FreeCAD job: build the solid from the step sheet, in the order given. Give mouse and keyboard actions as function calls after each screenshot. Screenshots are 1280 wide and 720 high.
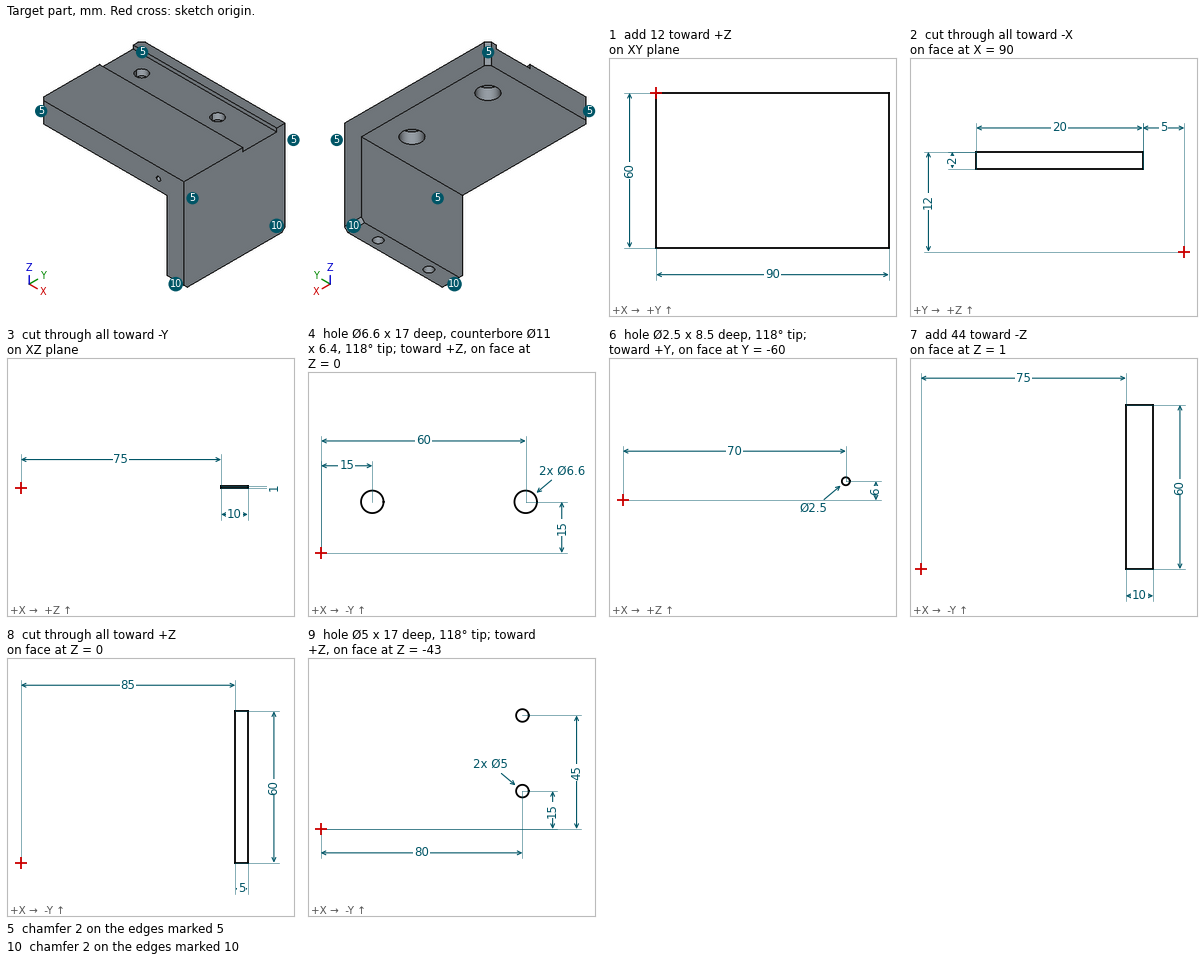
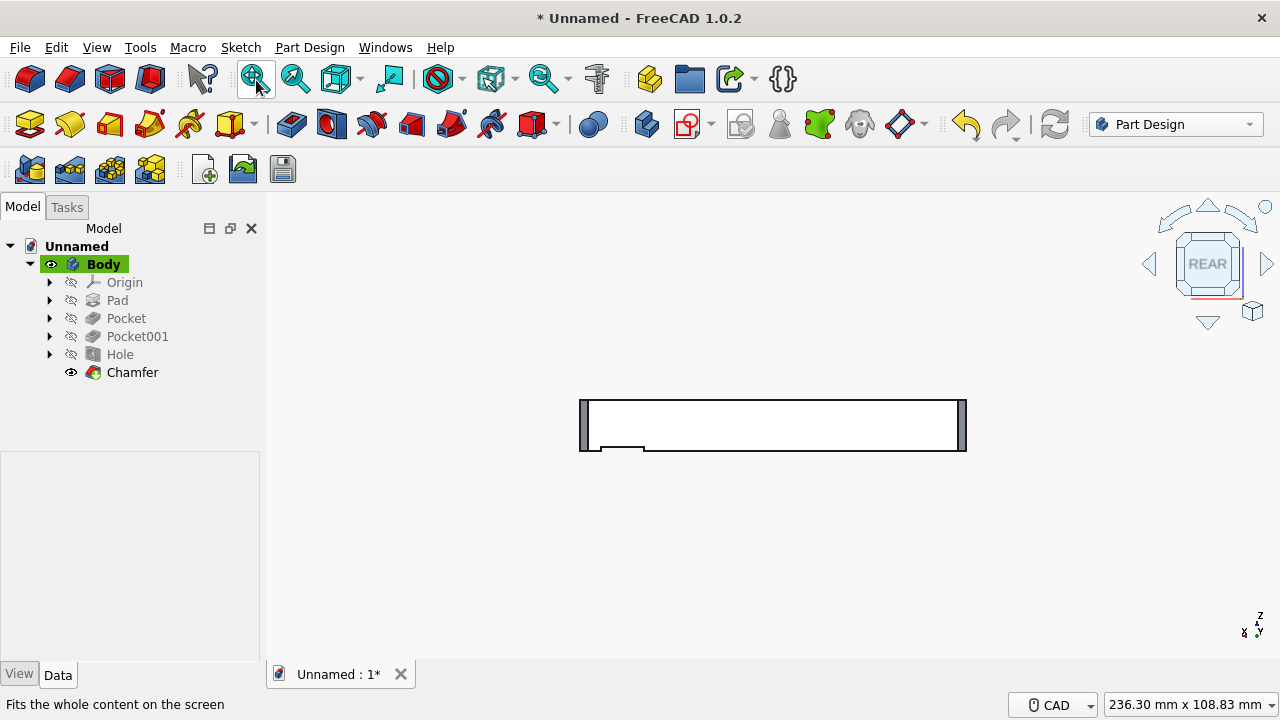
key(0)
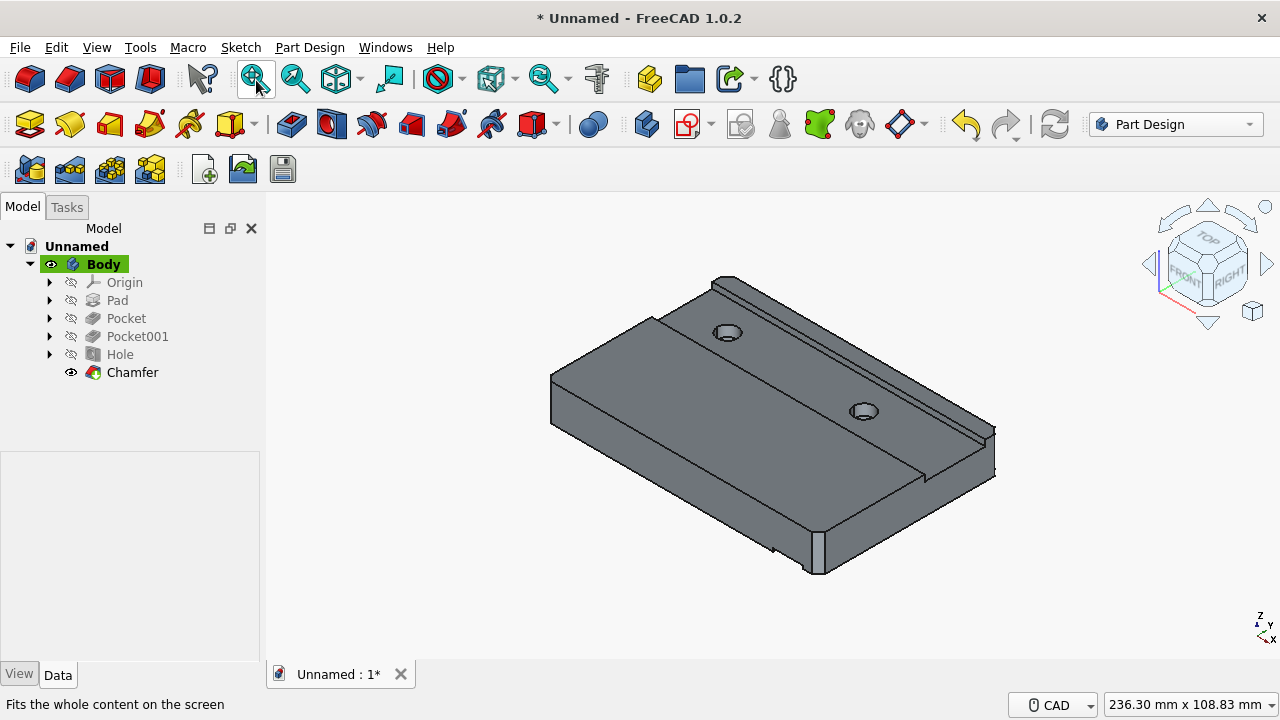
click(757, 520)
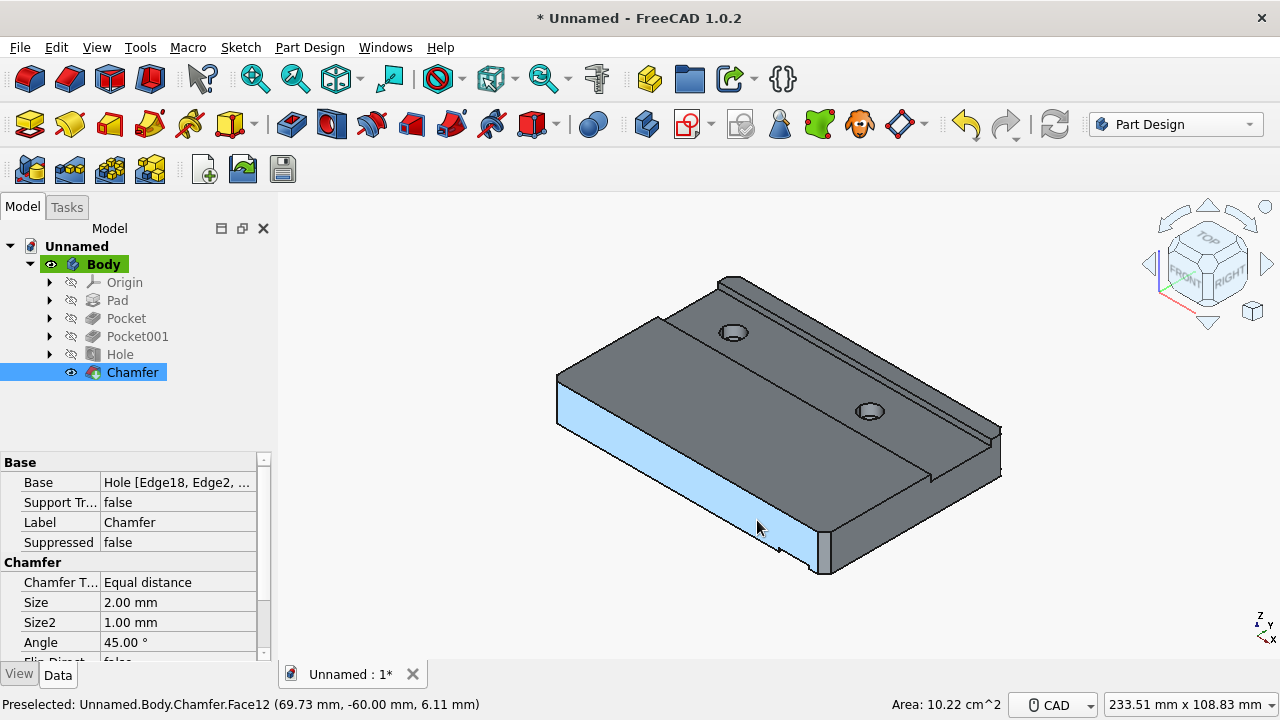
click(688, 124)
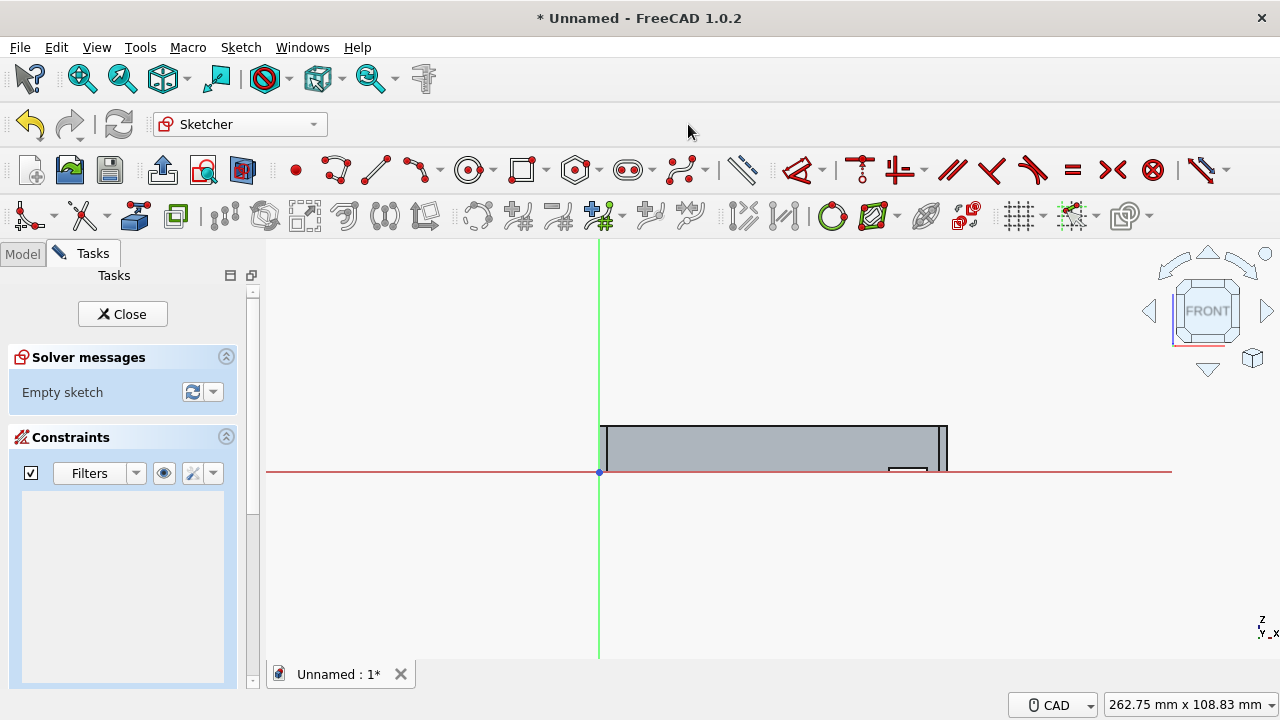
scroll(878, 449, up, 15)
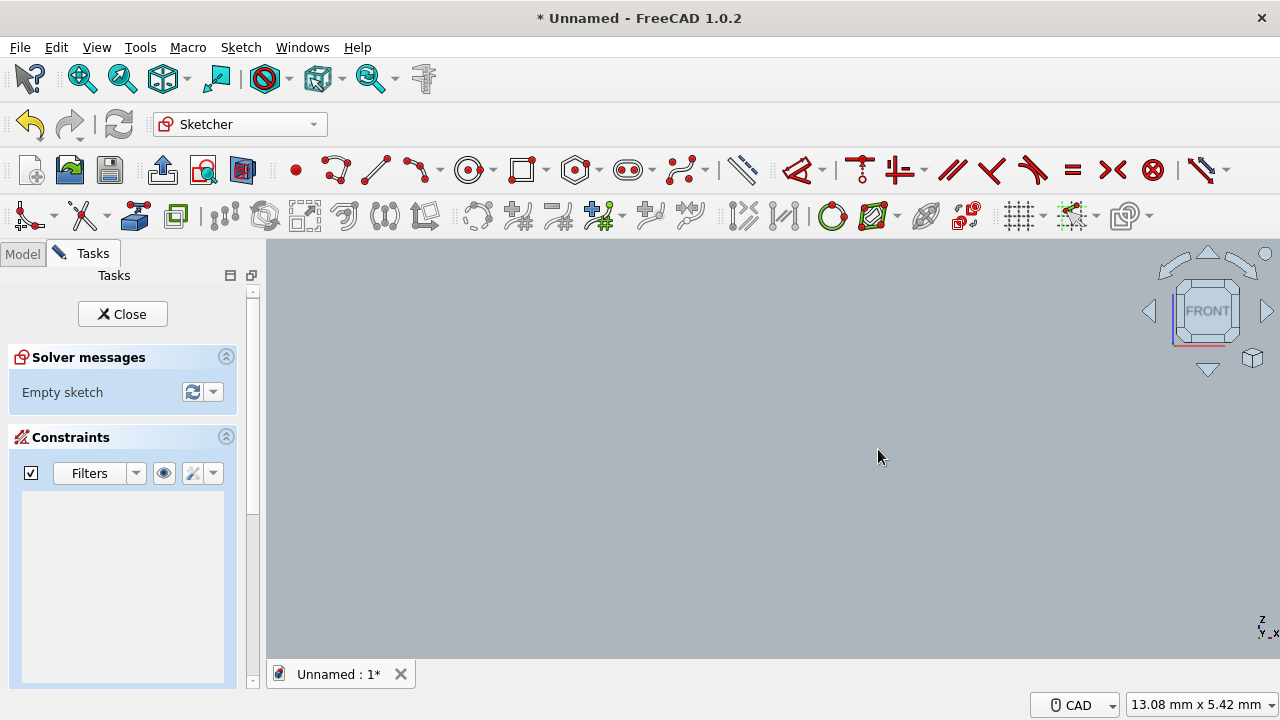
click(470, 170)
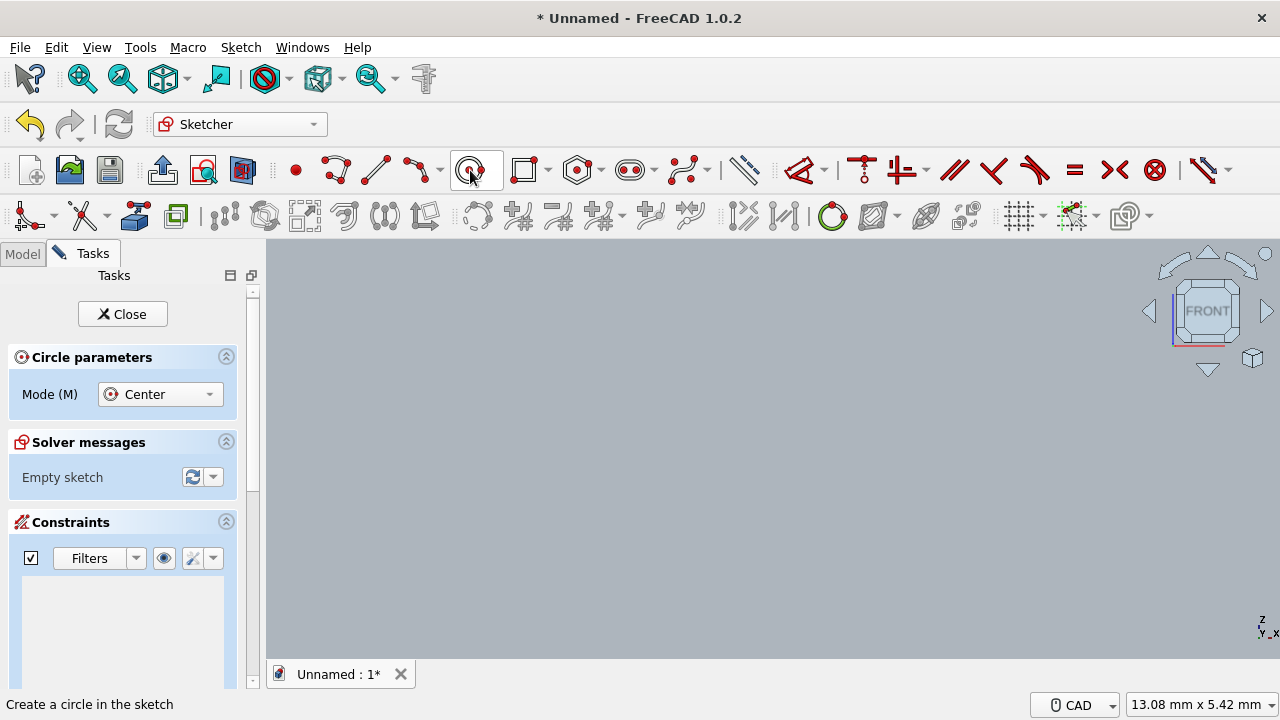
click(695, 439)
click(764, 371)
key(Escape)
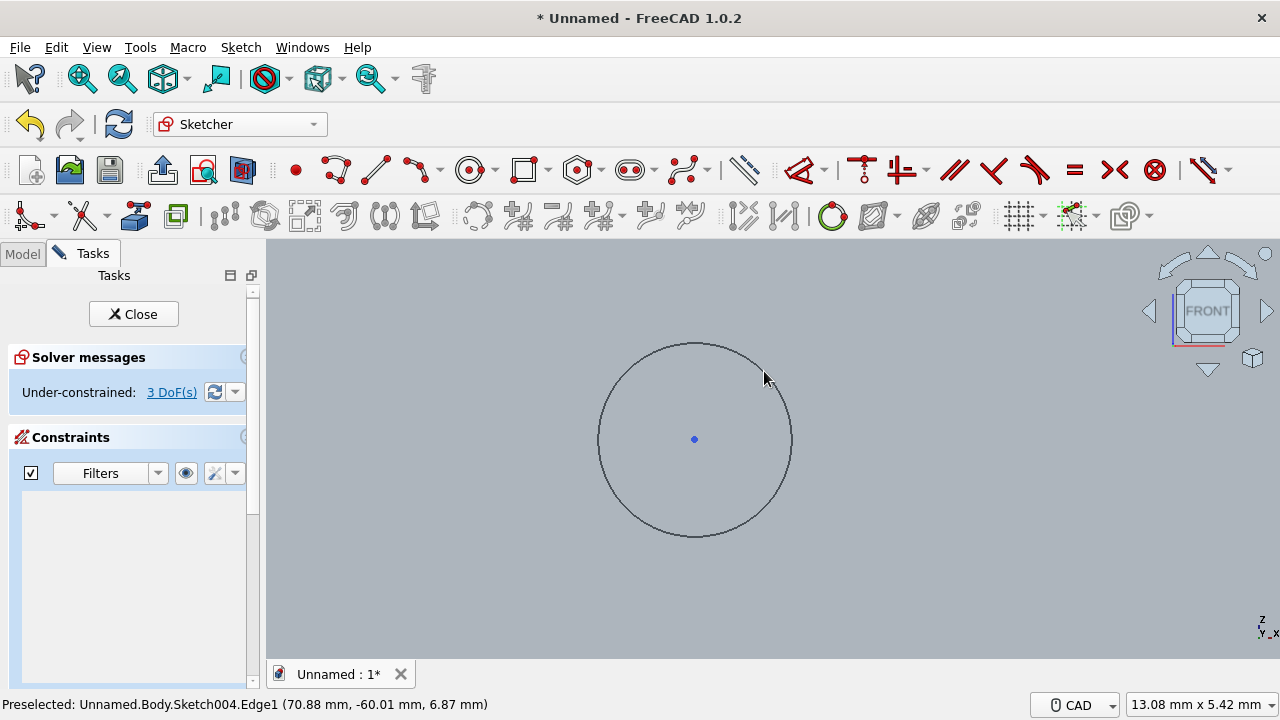
key(d)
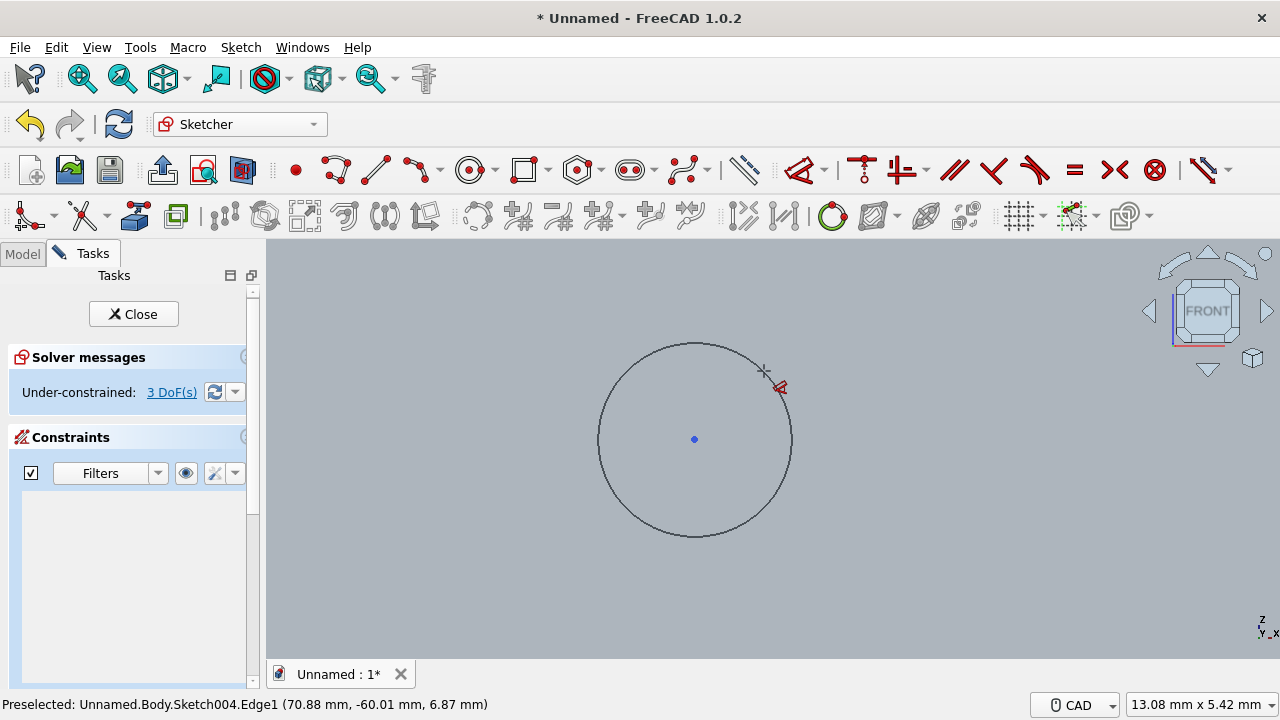
click(763, 371)
click(785, 348)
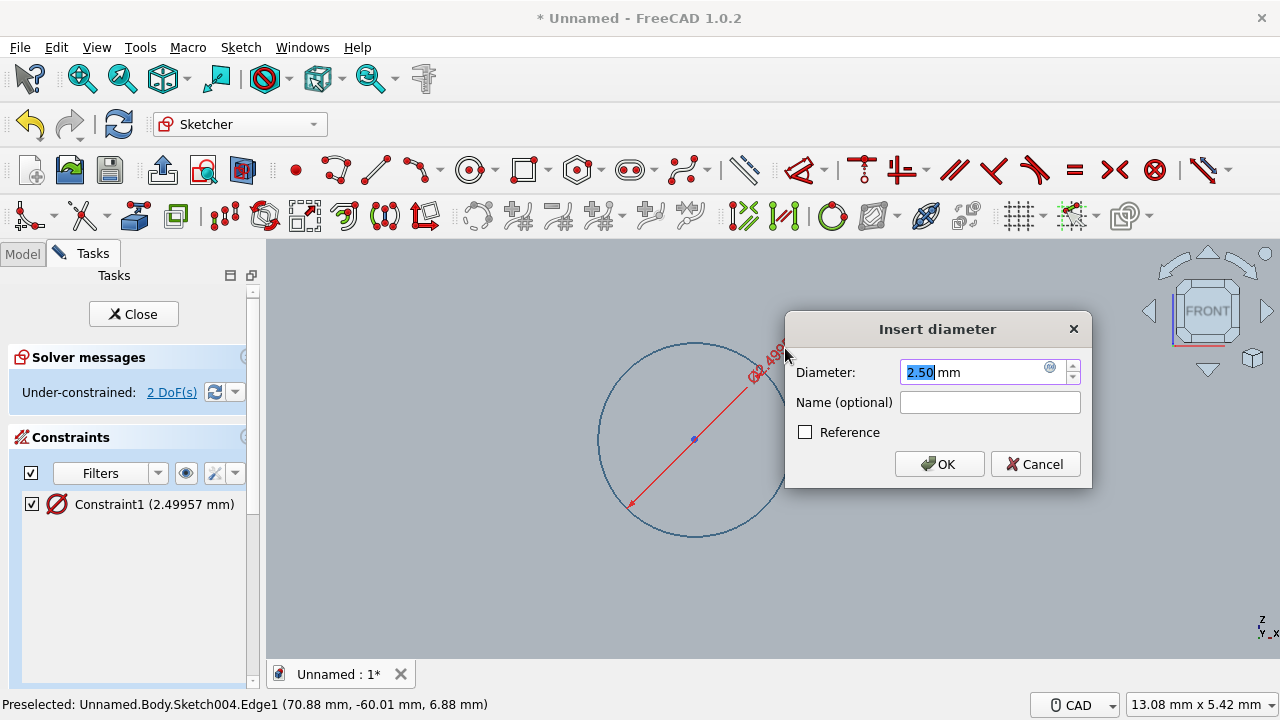
text(2.5)
key(Return)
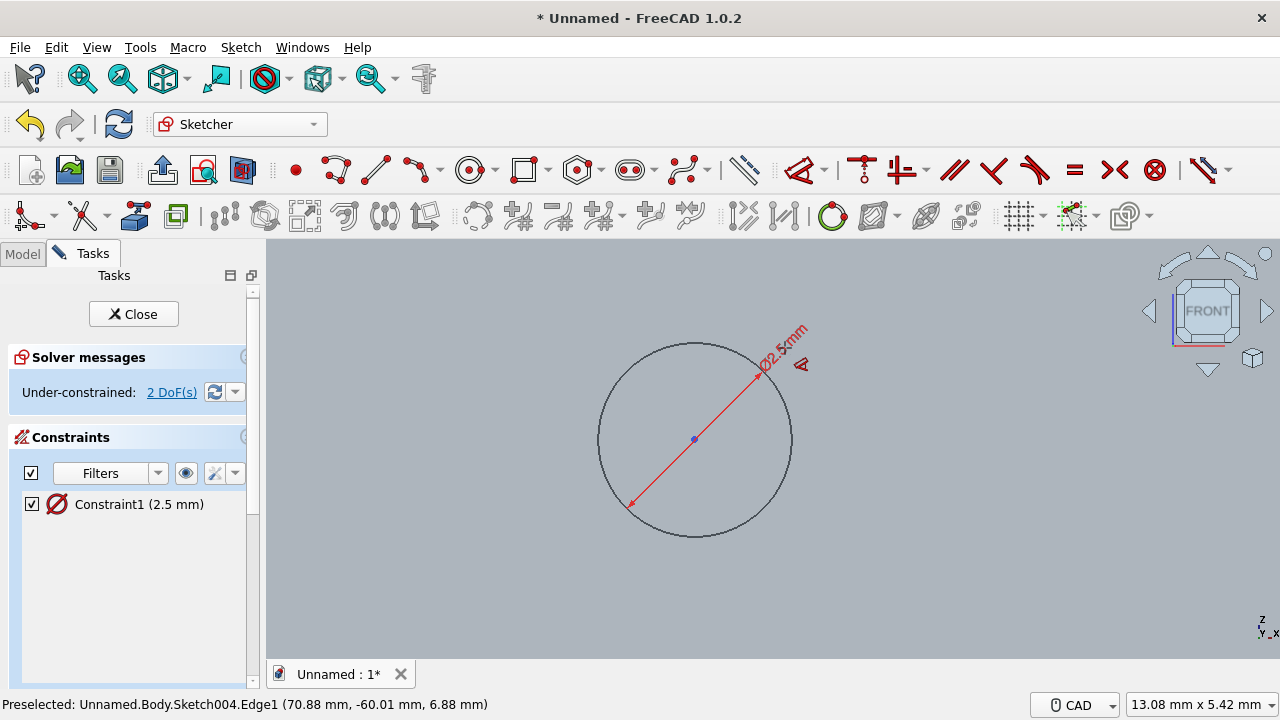
click(695, 440)
click(729, 492)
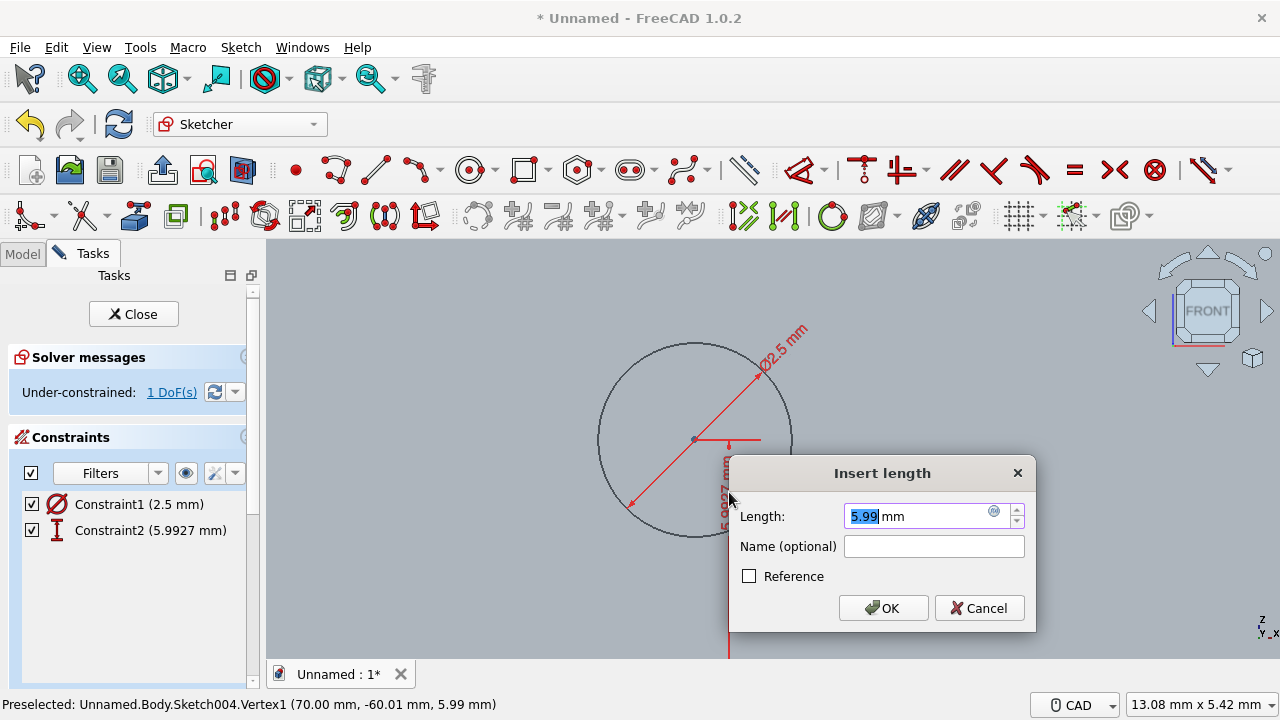
text(6)
key(Return)